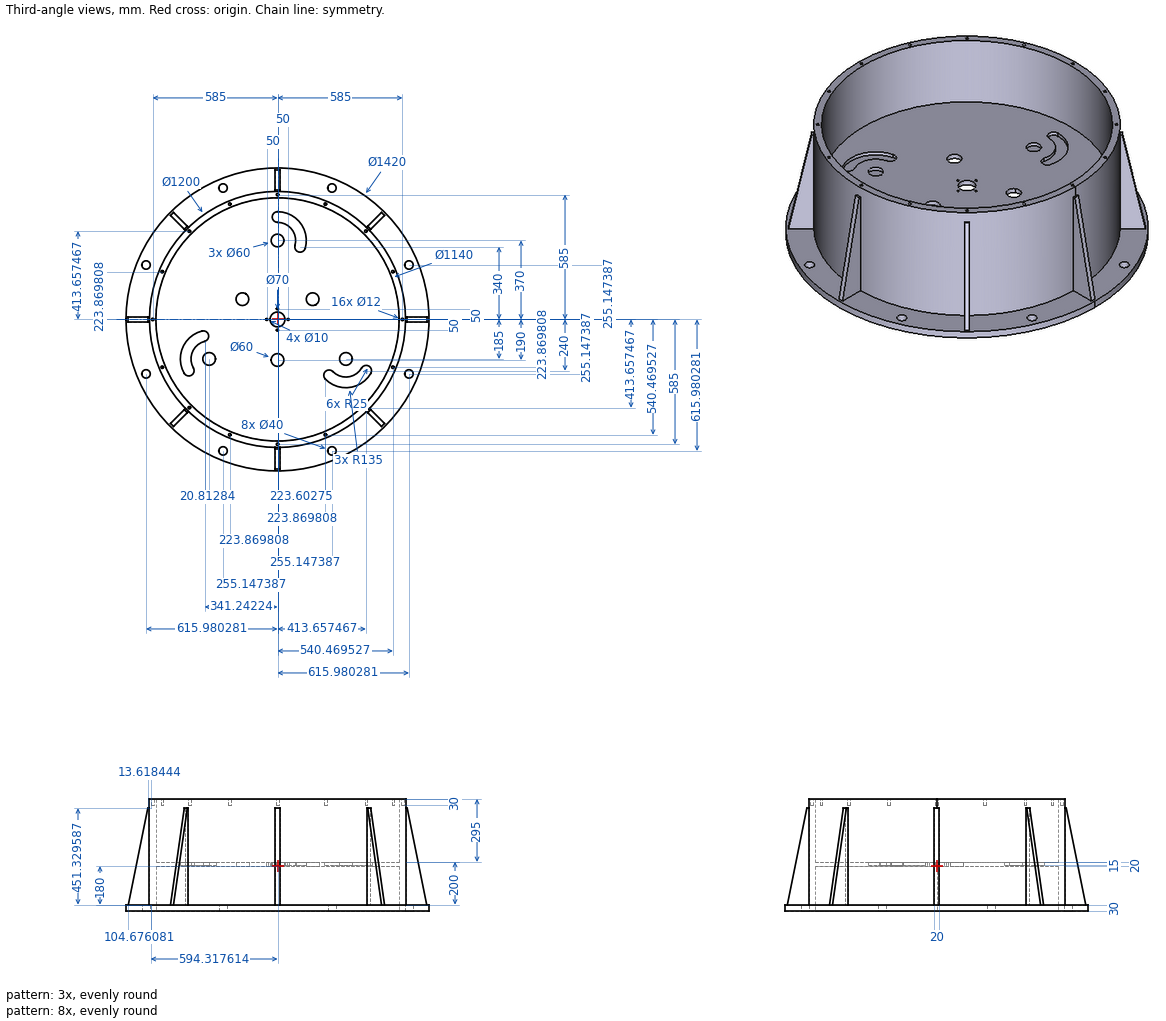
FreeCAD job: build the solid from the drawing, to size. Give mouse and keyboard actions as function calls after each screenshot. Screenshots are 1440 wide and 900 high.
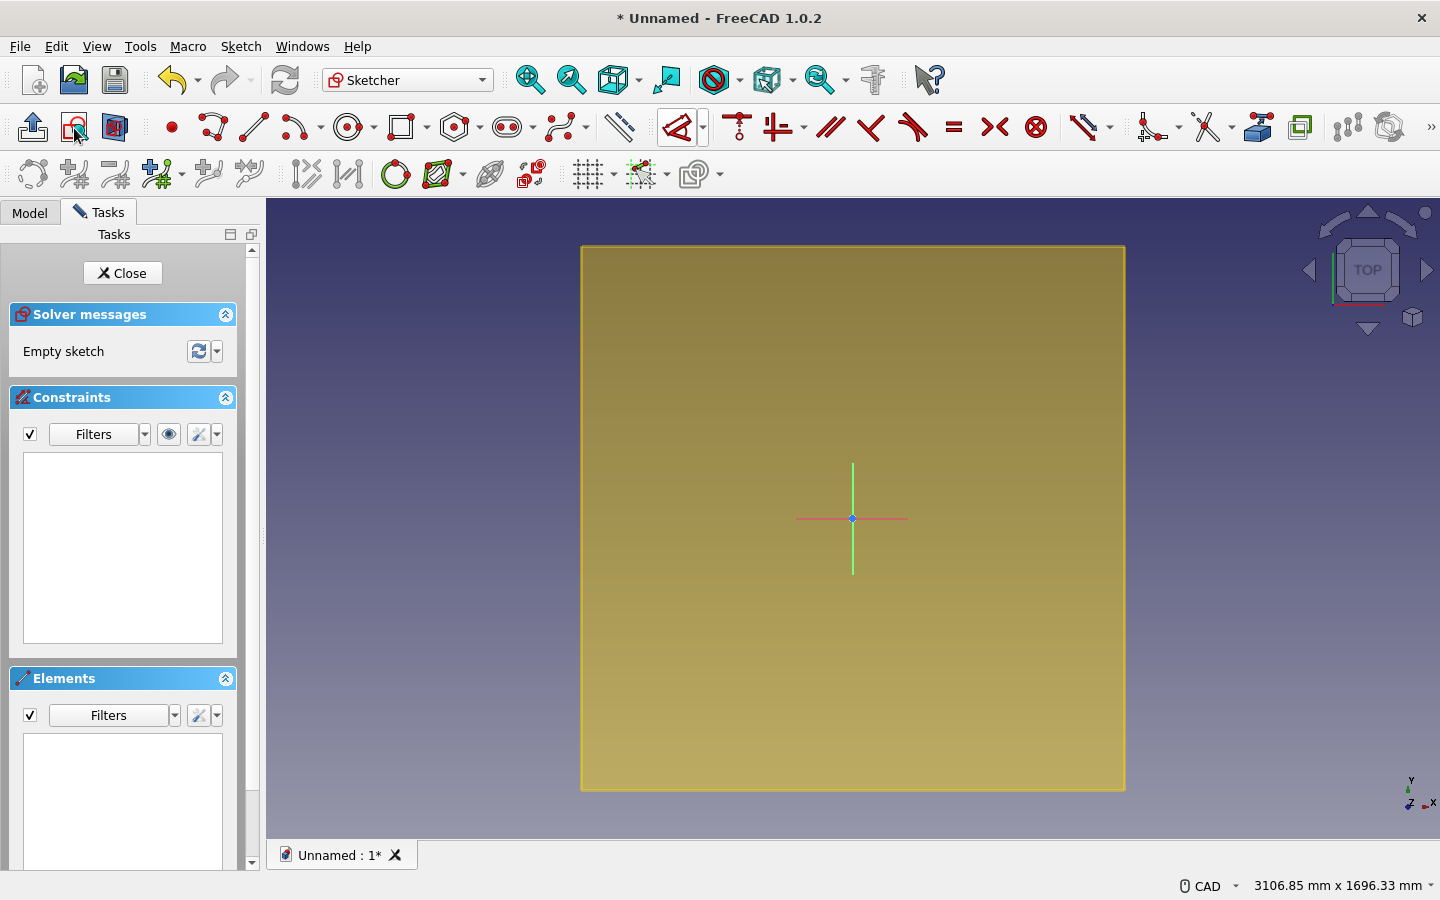
click(348, 128)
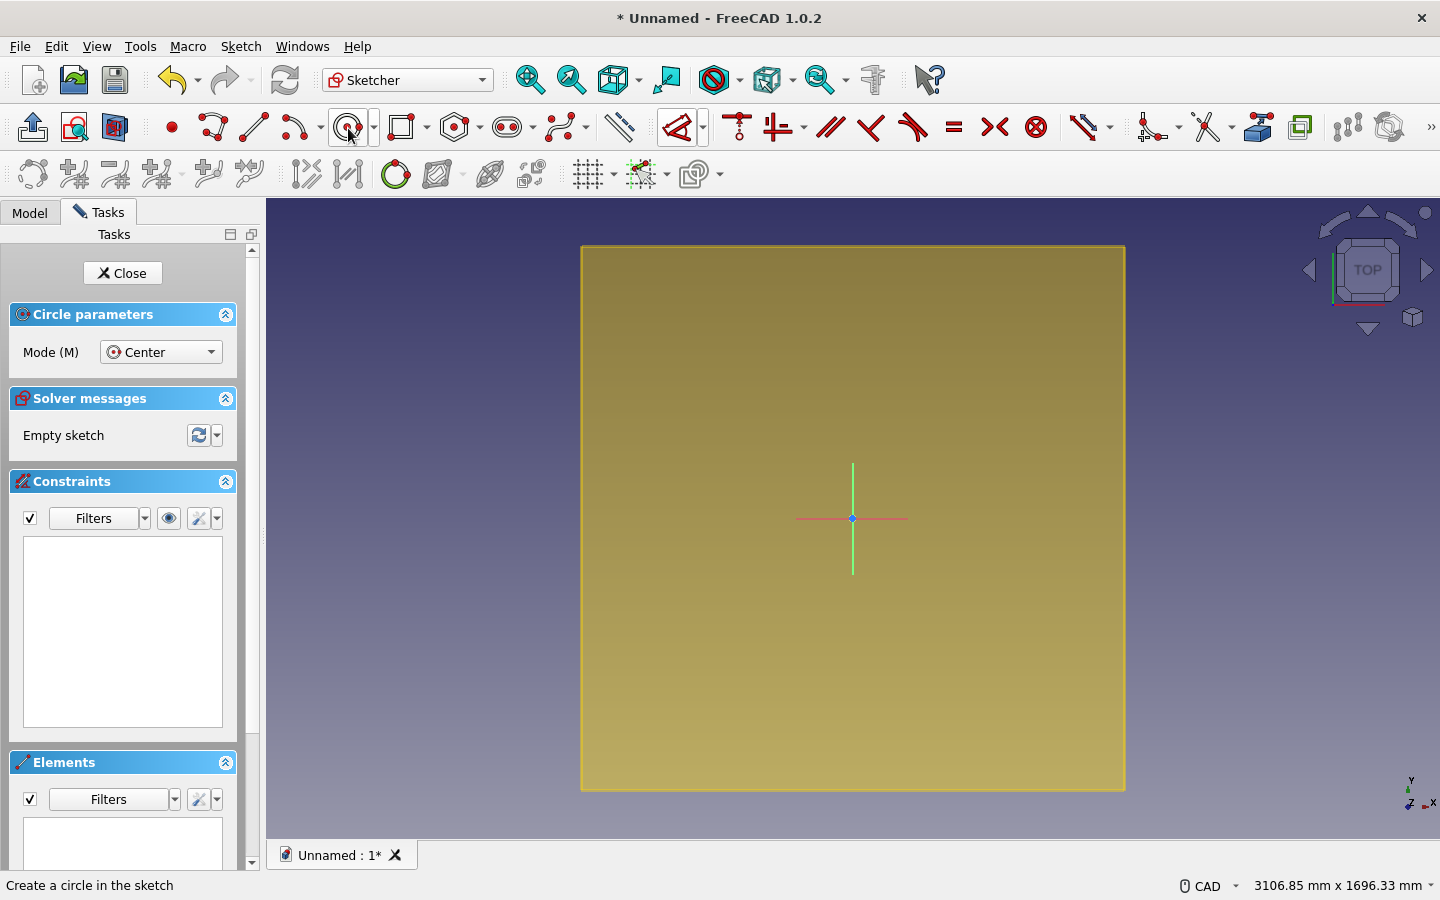
click(853, 518)
move(1013, 358)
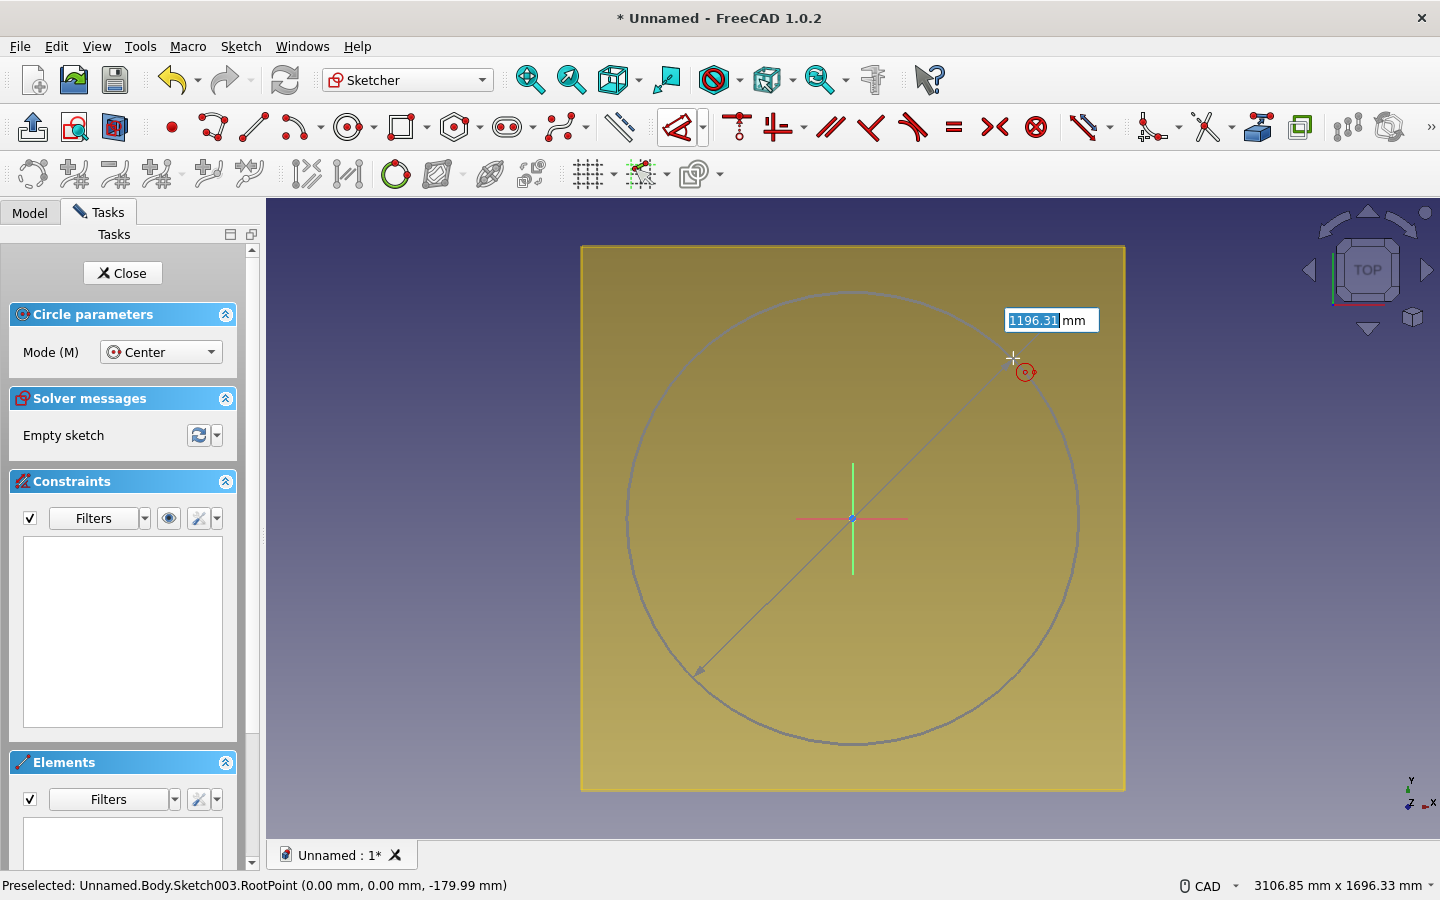
text(1200)
key(Return)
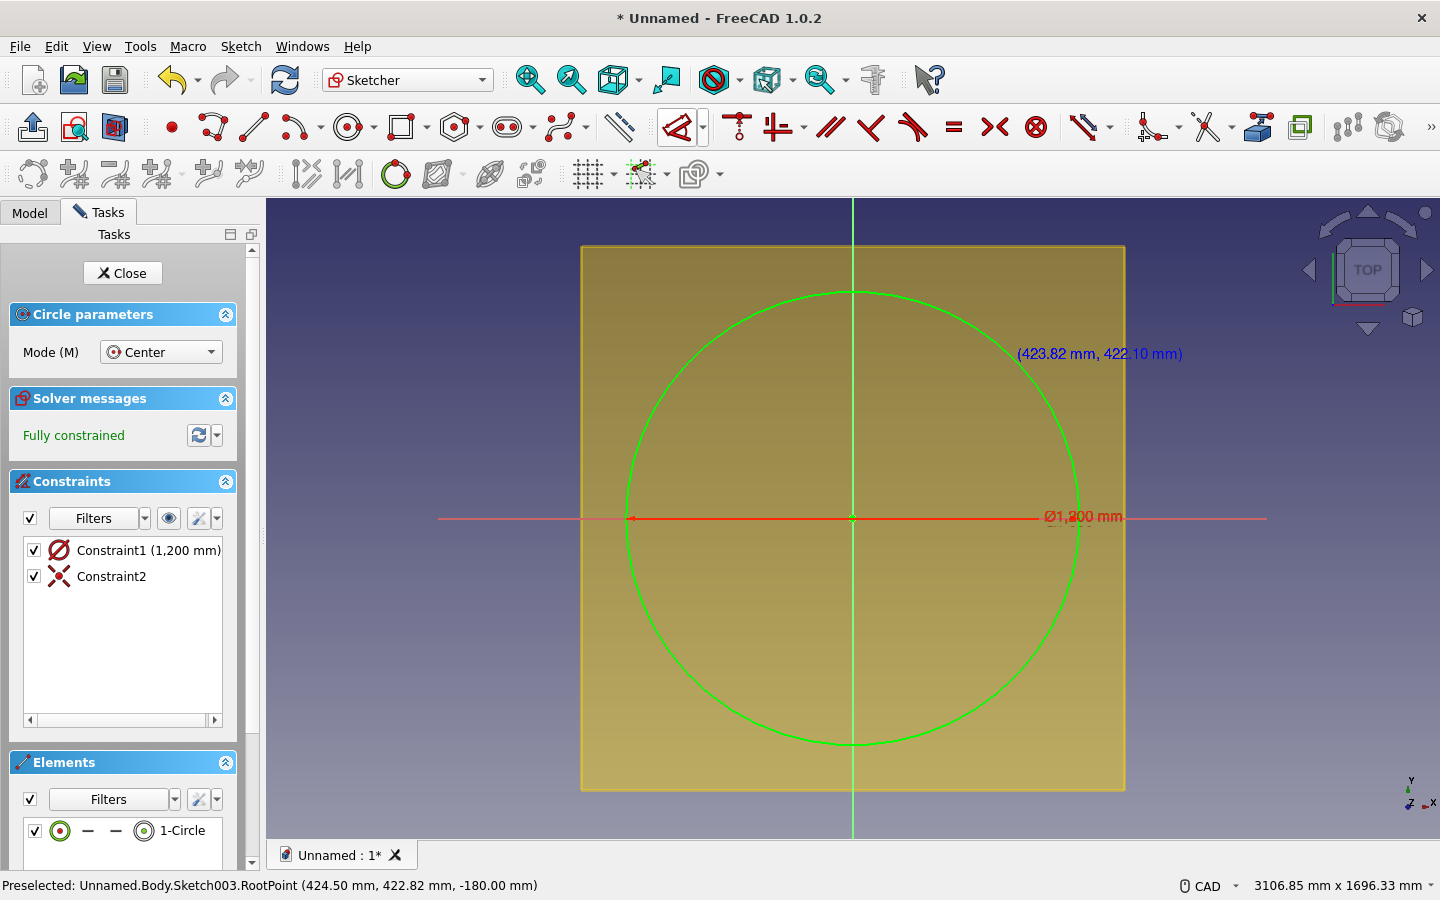
click(853, 518)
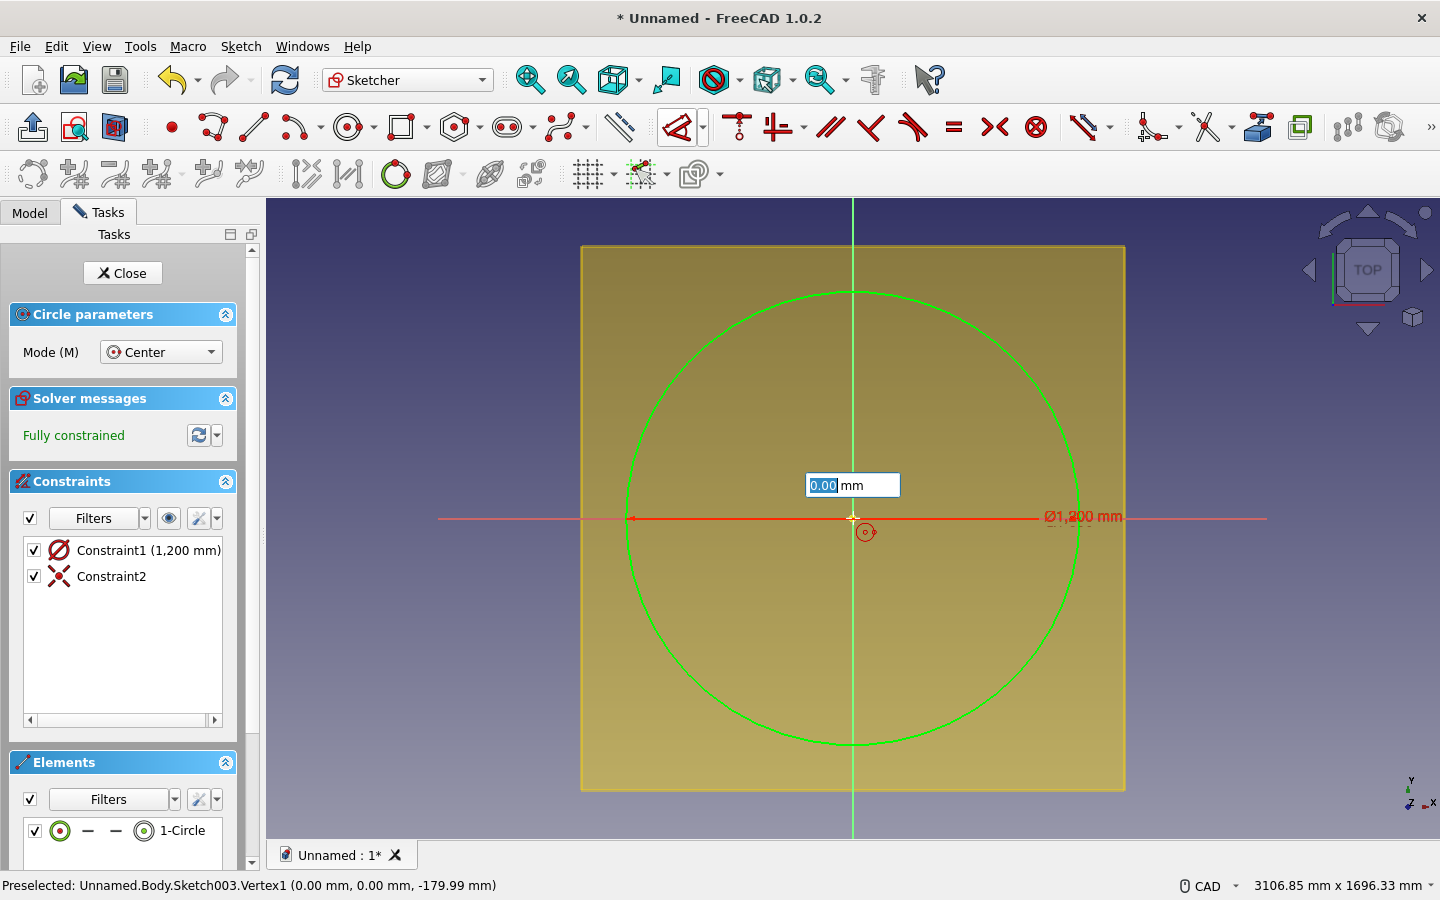
scroll(1005, 366, up, 2)
move(1005, 366)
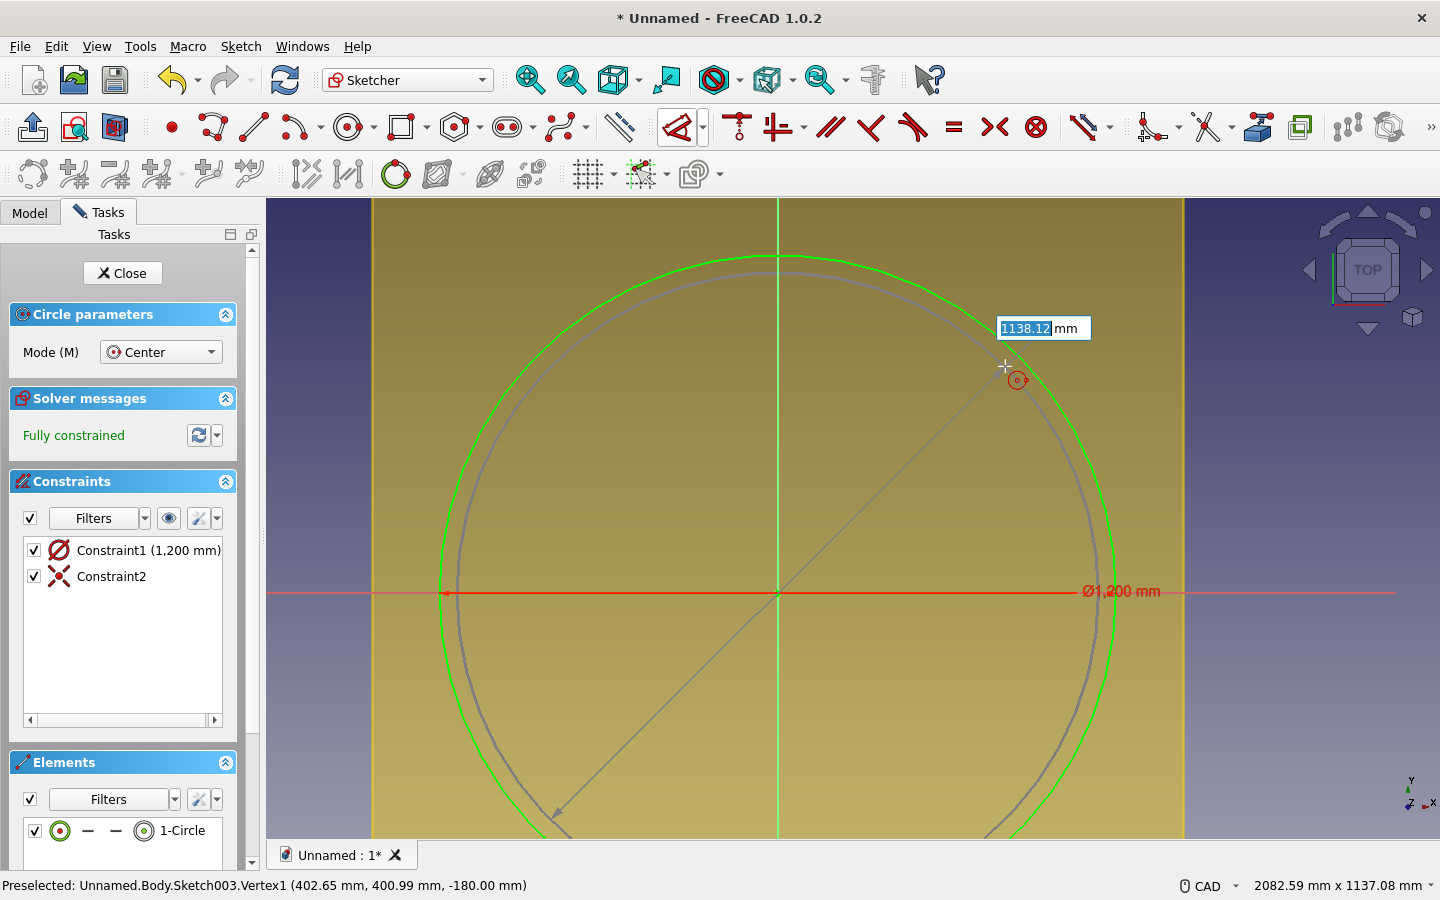
text(1140)
key(Return)
key(Escape)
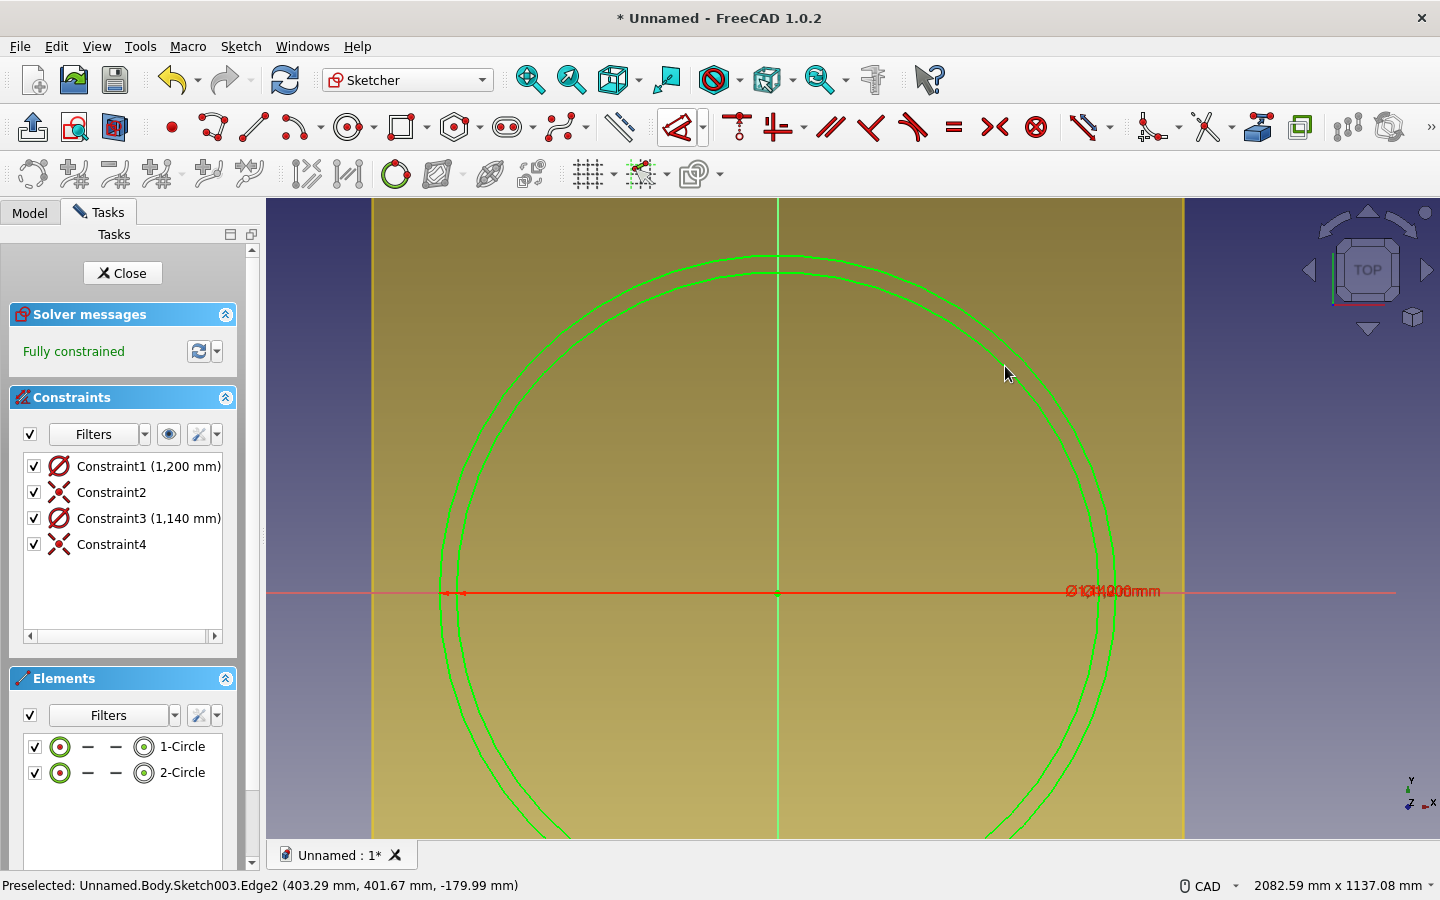
click(123, 273)